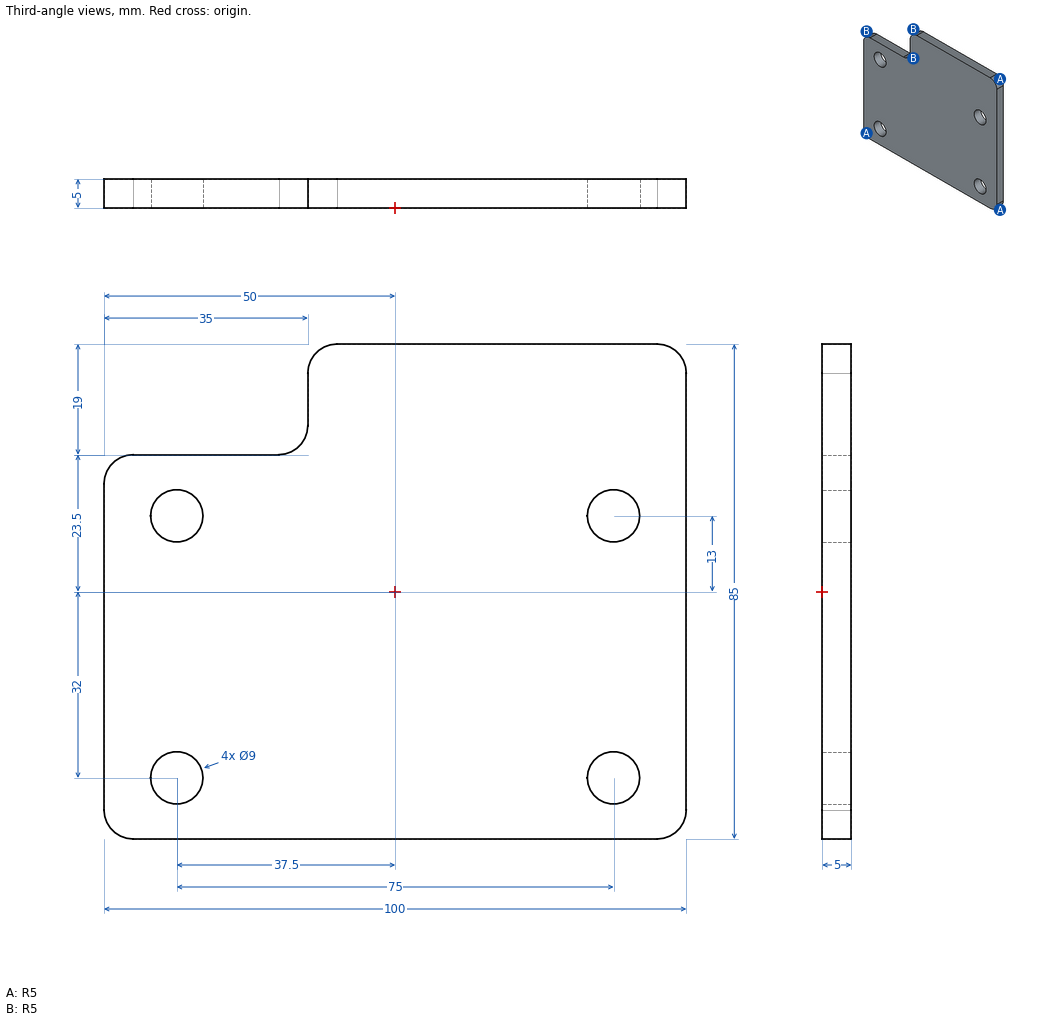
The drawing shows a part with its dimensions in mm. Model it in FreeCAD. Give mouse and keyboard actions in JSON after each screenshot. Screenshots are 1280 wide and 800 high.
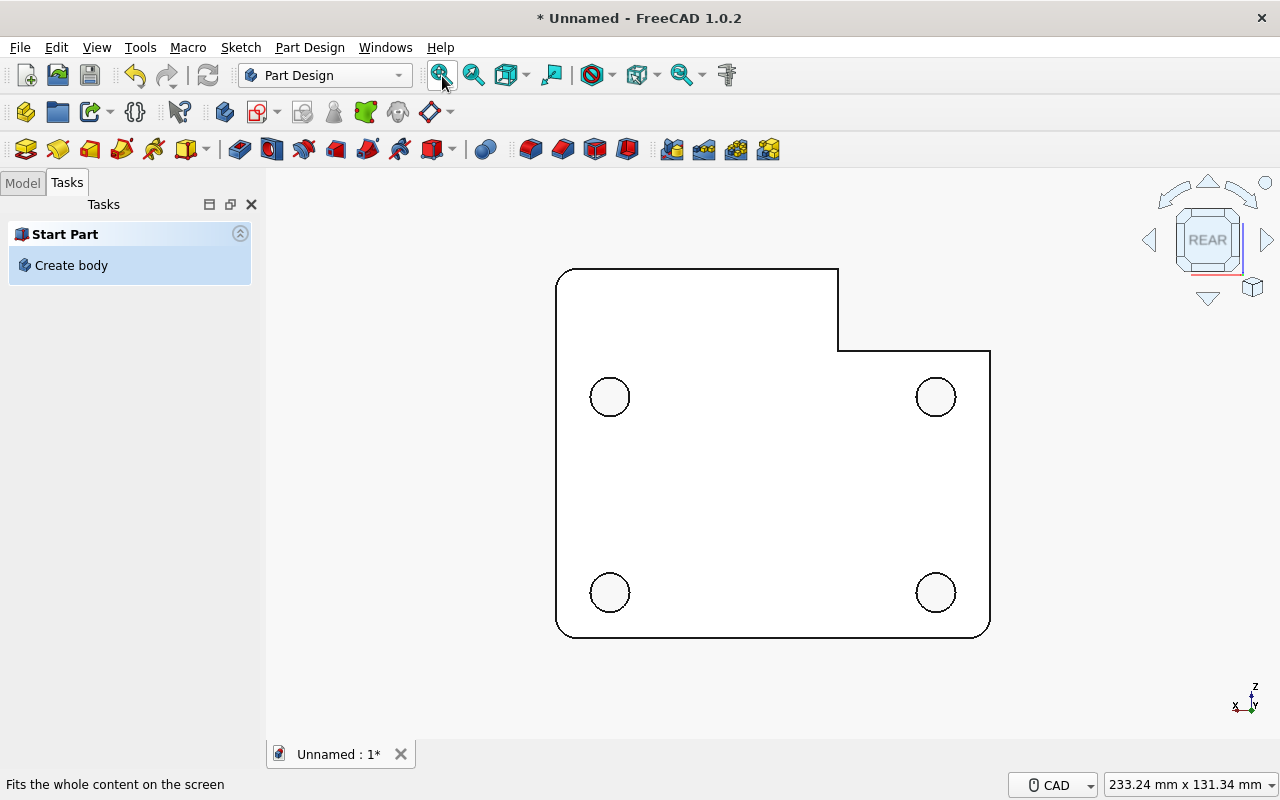
{"action": "key", "text": "0"}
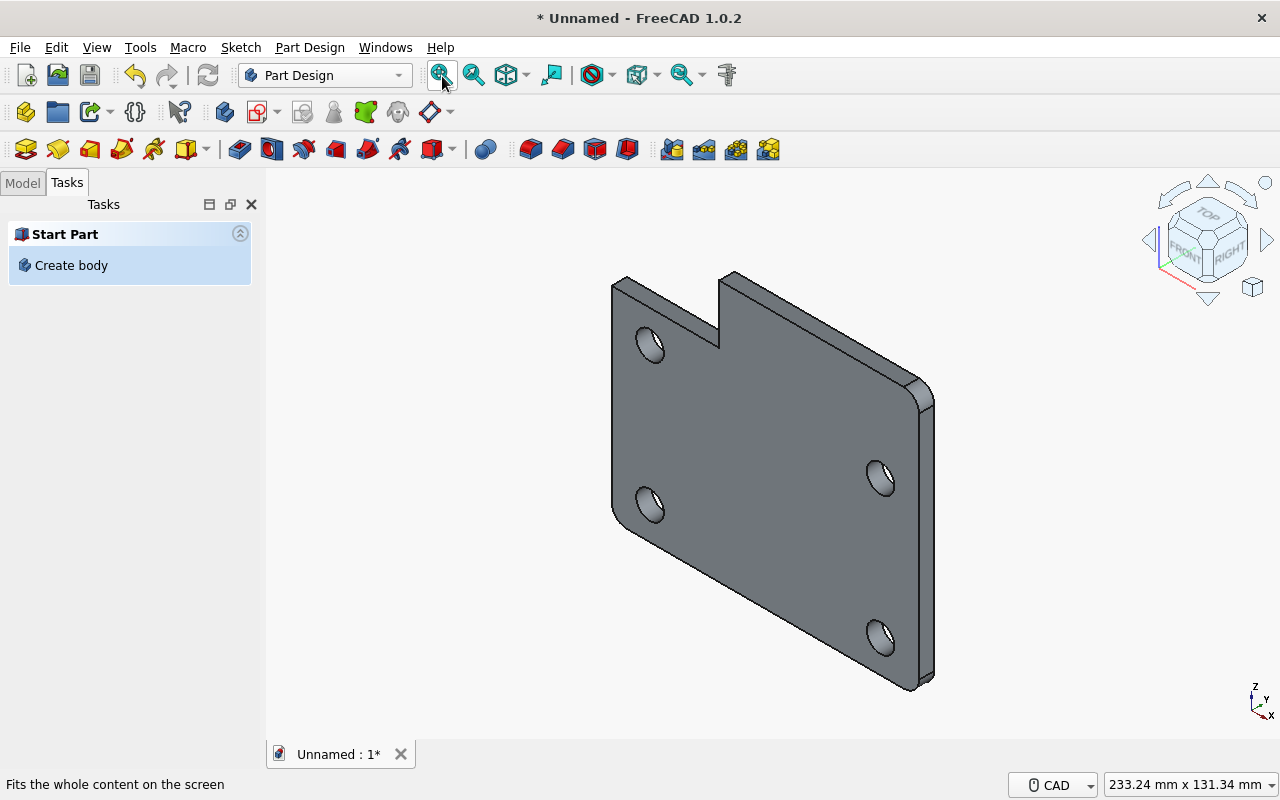
{"action": "scroll", "coordinate": [619, 280], "scroll_direction": "up", "scroll_amount": 4}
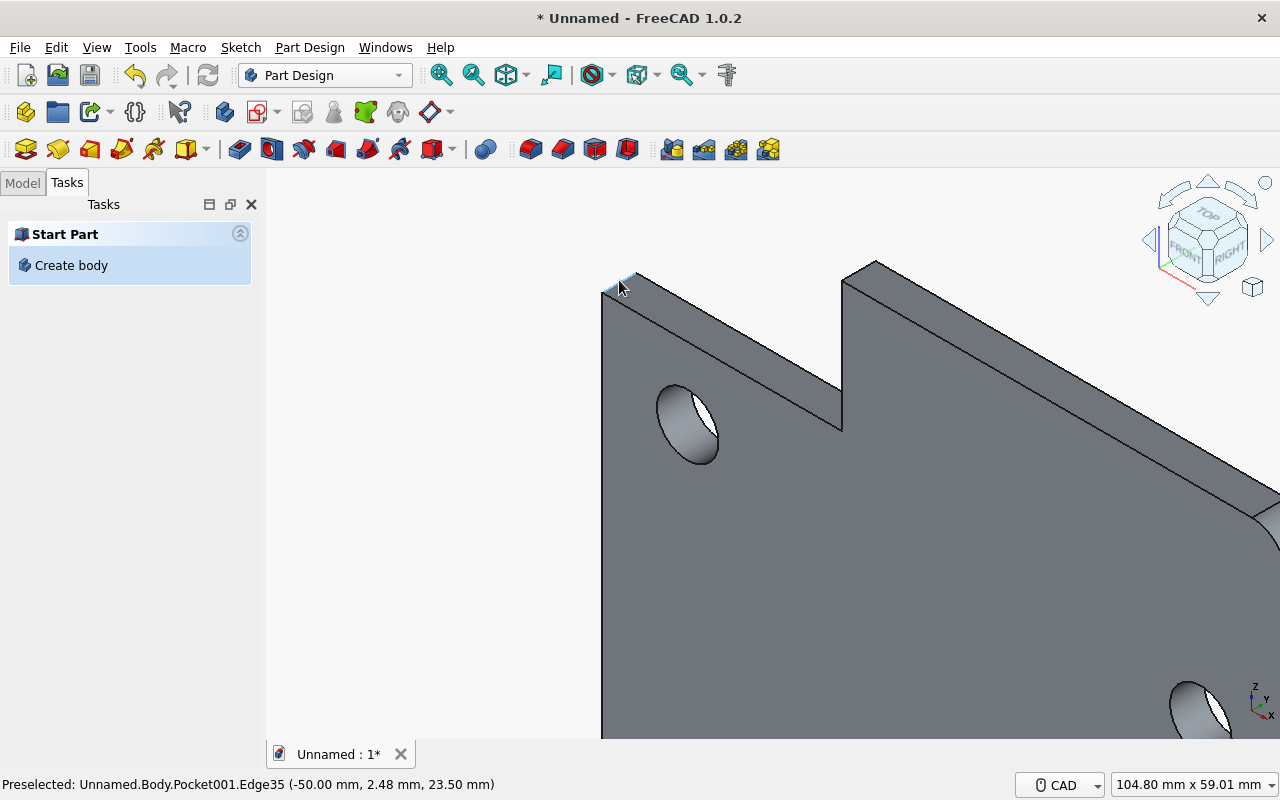
{"action": "key", "text": "v f"}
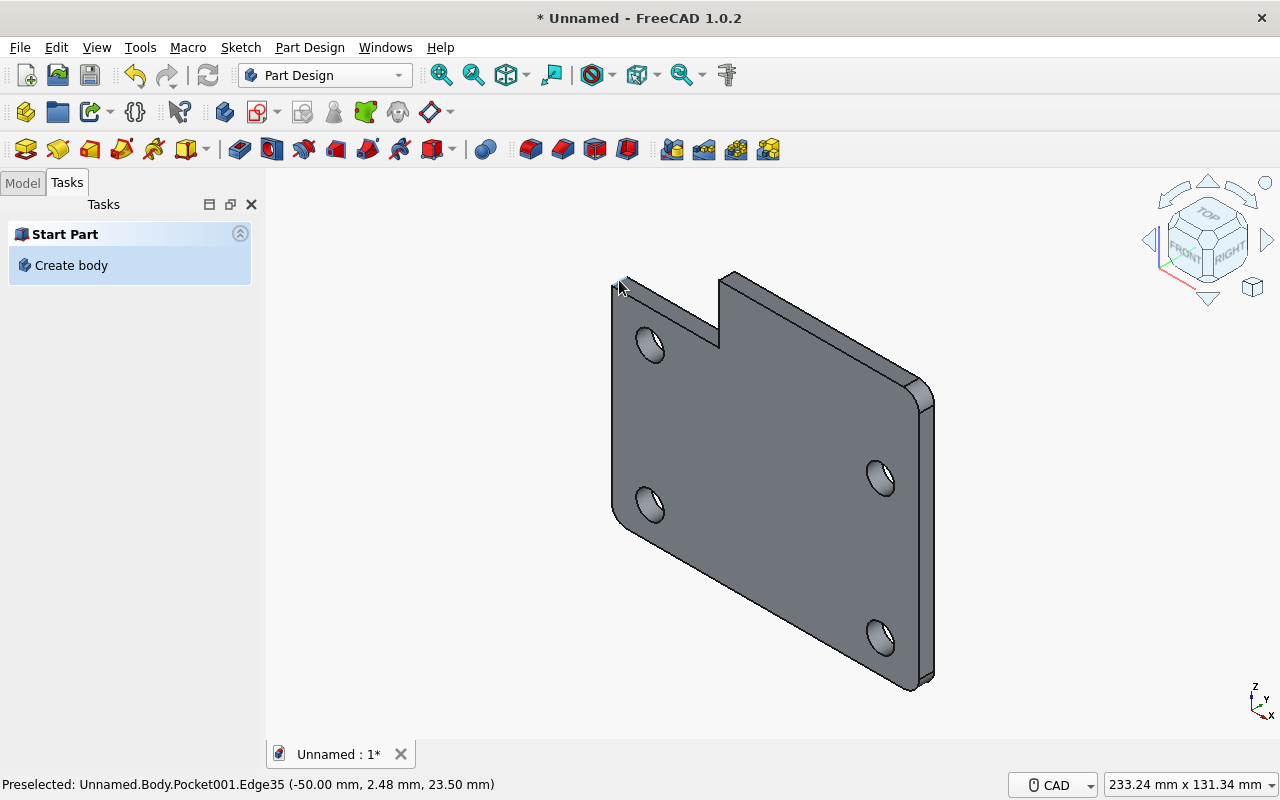
{"action": "key", "text": "2"}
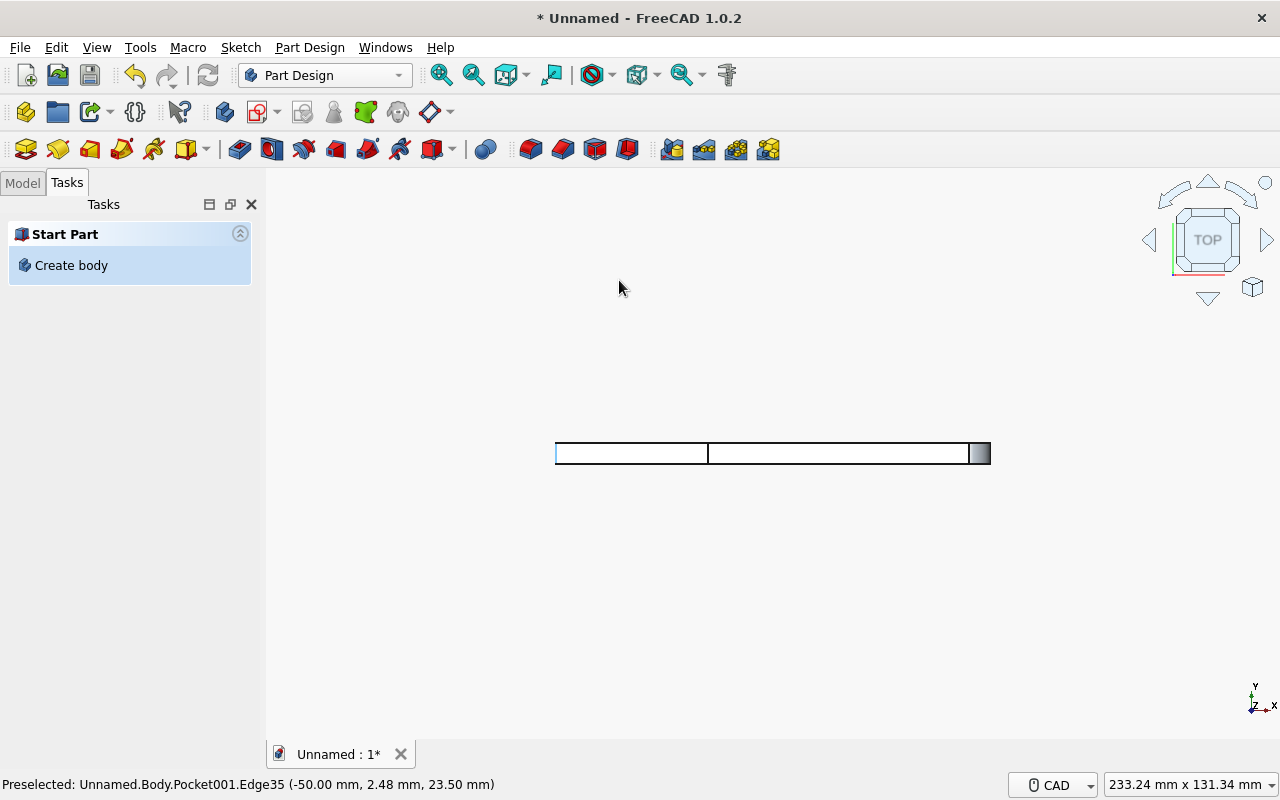
{"action": "left_click", "coordinate": [442, 76]}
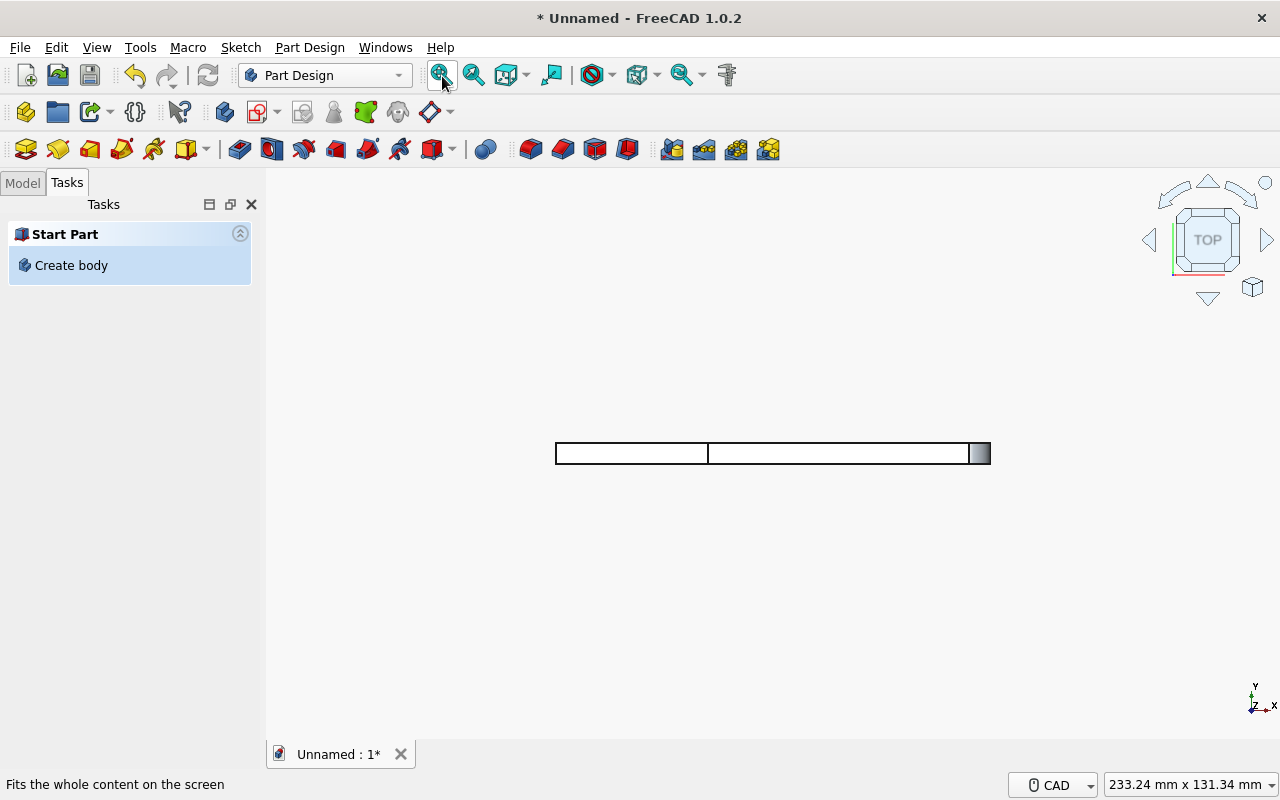
{"action": "left_click", "coordinate": [556, 452]}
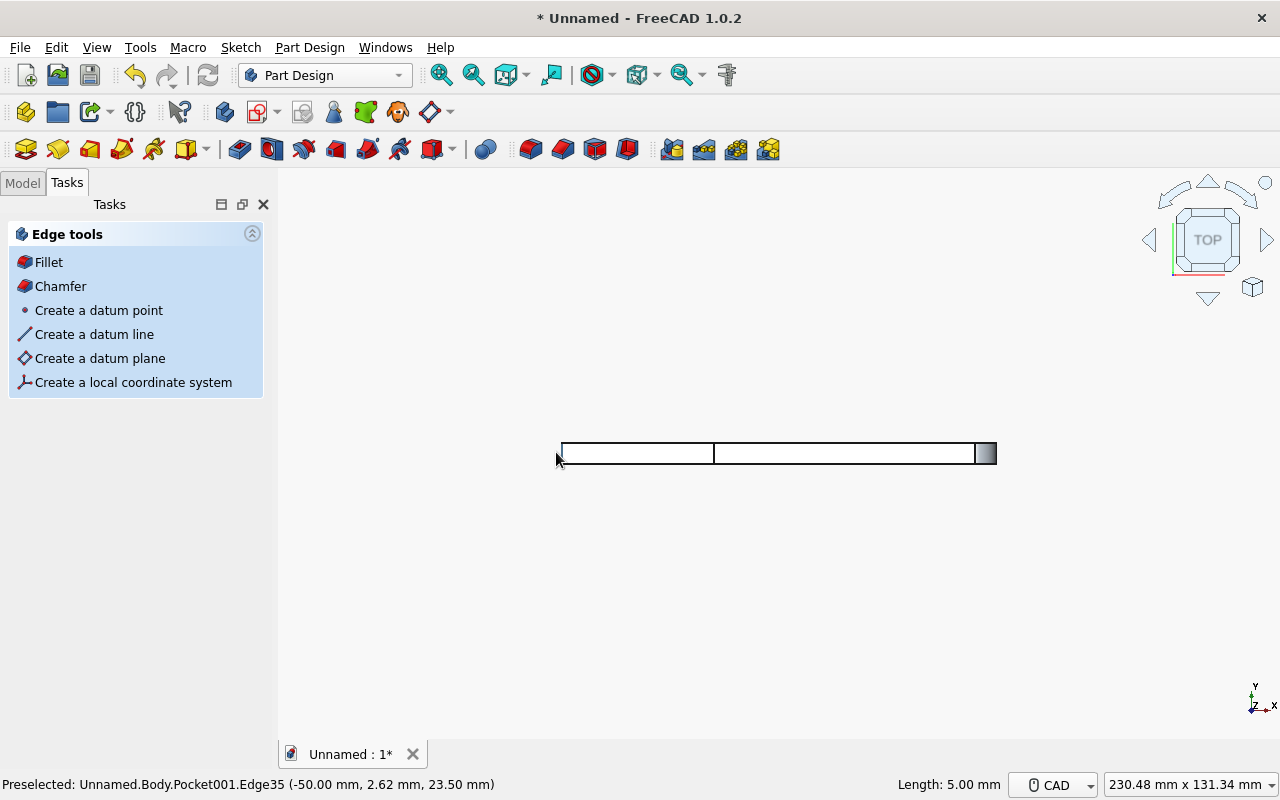
{"action": "left_click", "coordinate": [714, 452], "text": "ctrl"}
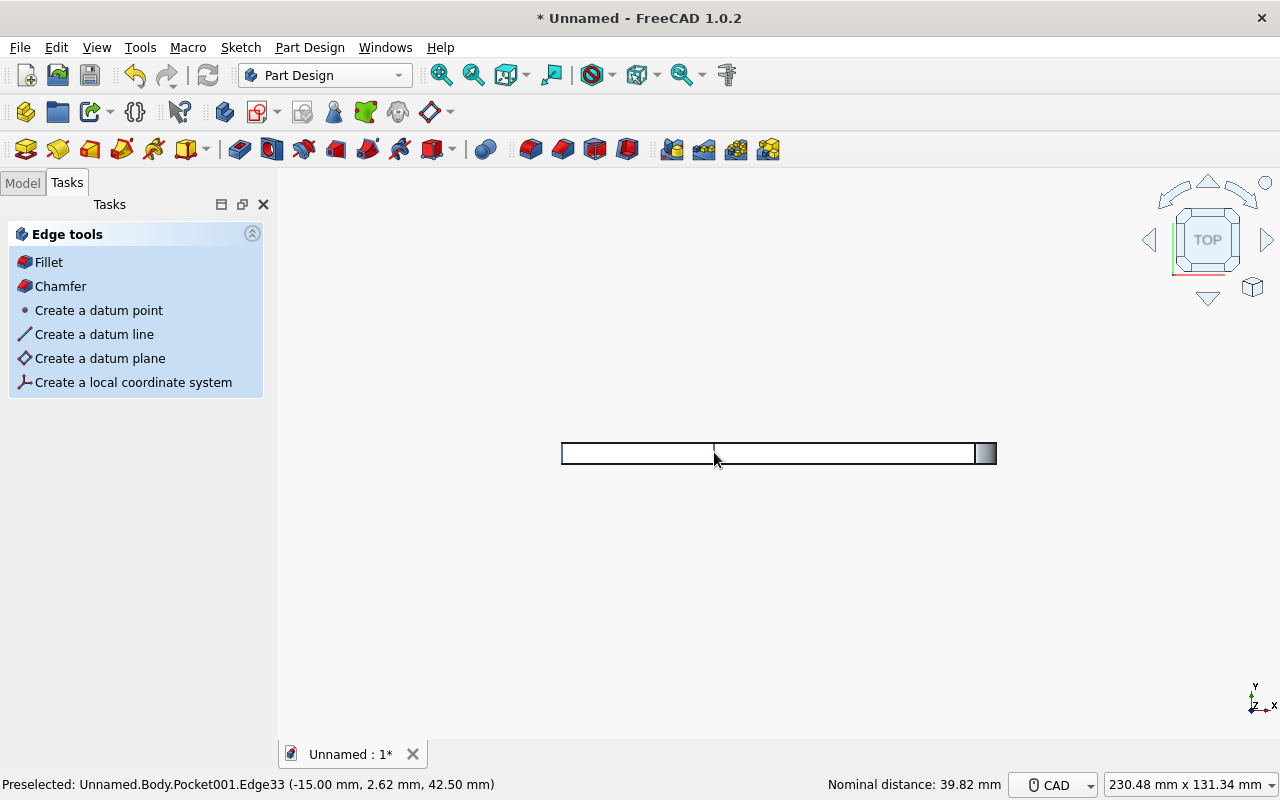
{"action": "scroll", "coordinate": [714, 452], "scroll_direction": "up", "scroll_amount": 4}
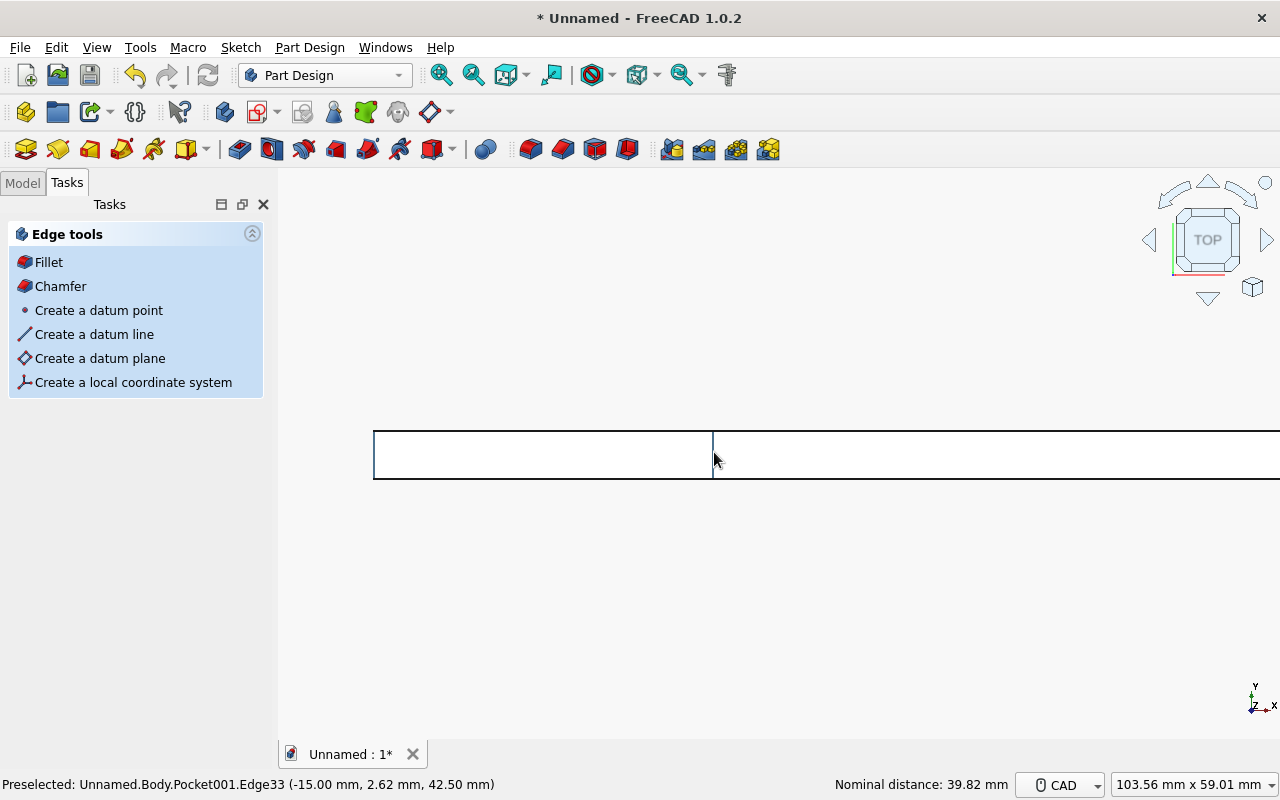
{"action": "left_click", "coordinate": [442, 76]}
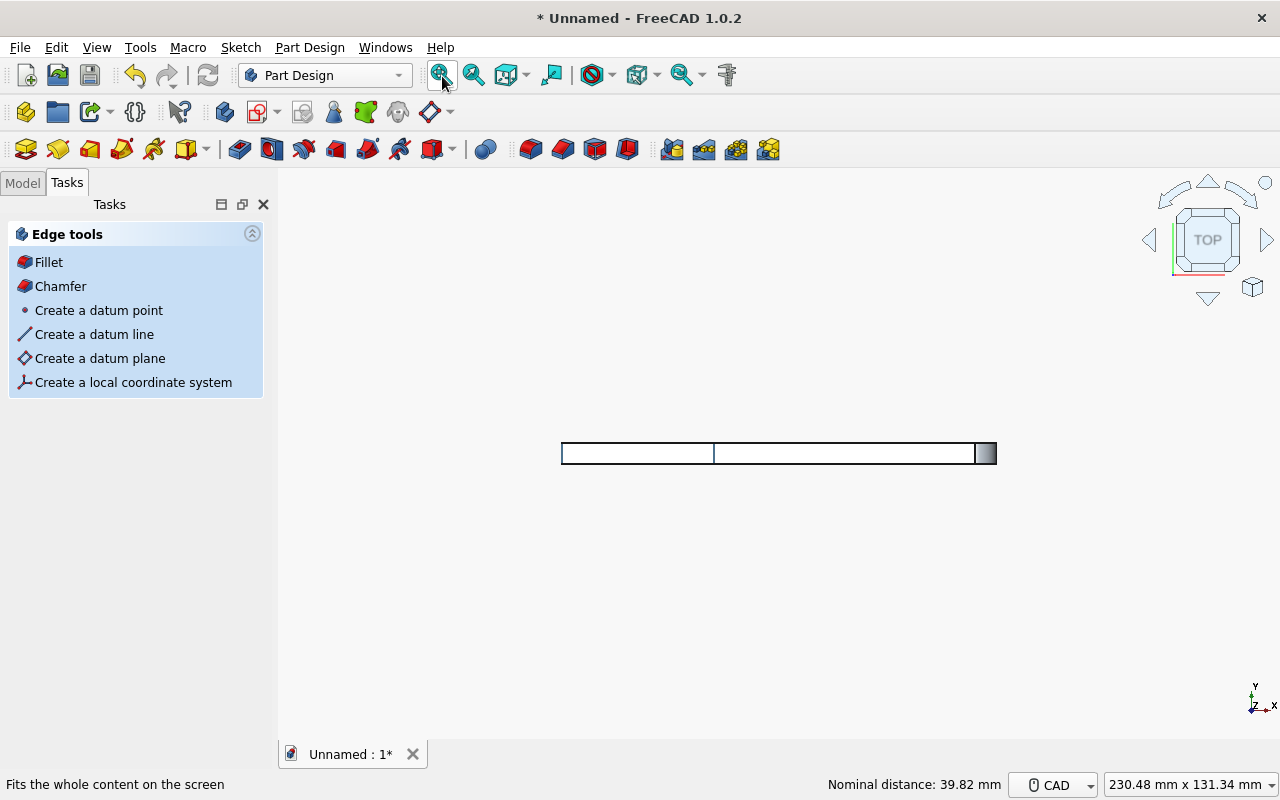
{"action": "key", "text": "1"}